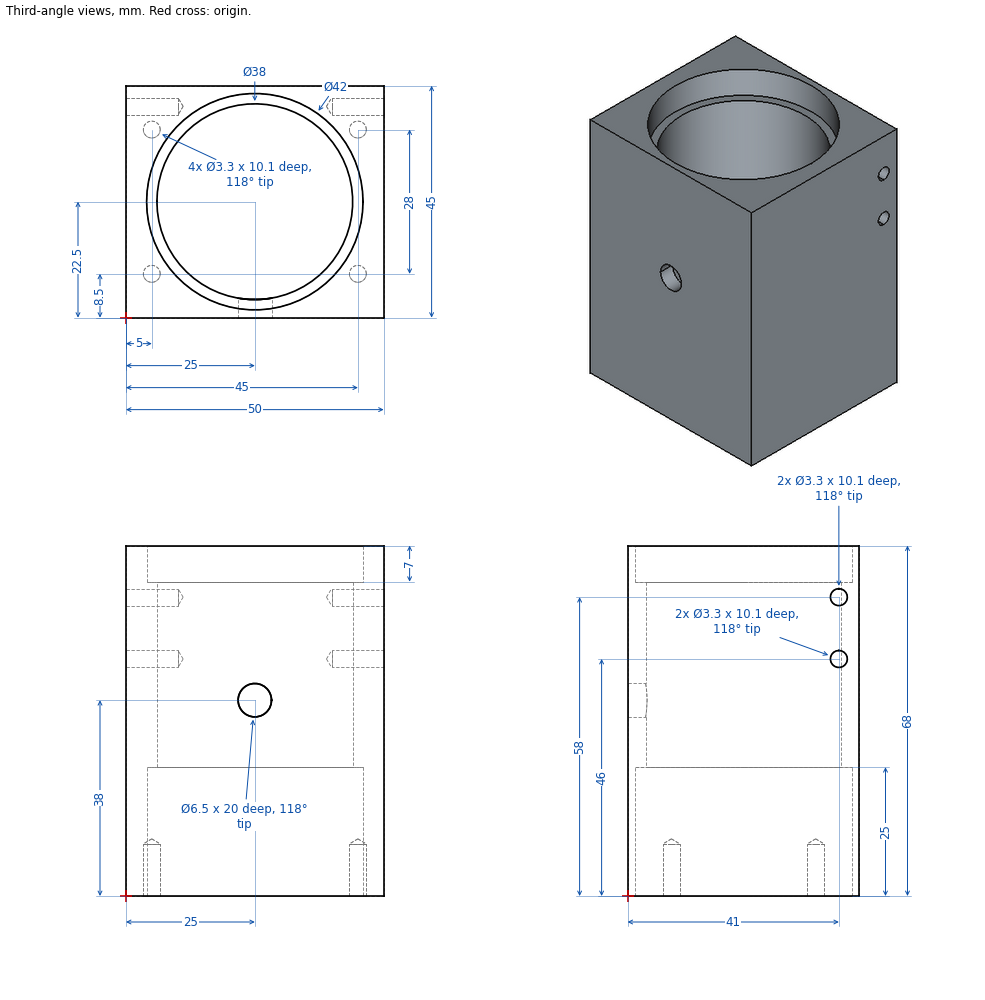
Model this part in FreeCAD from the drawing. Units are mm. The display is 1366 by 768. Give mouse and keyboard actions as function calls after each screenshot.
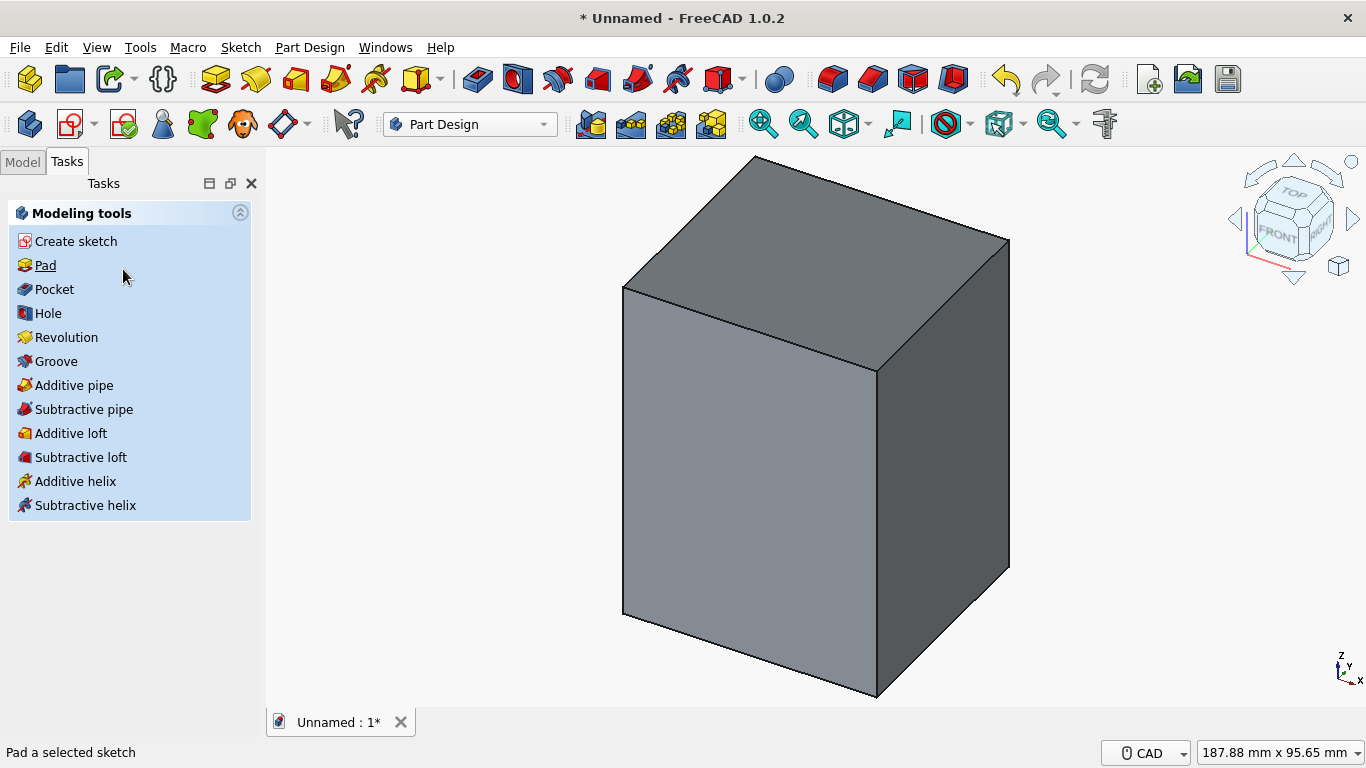
click(478, 80)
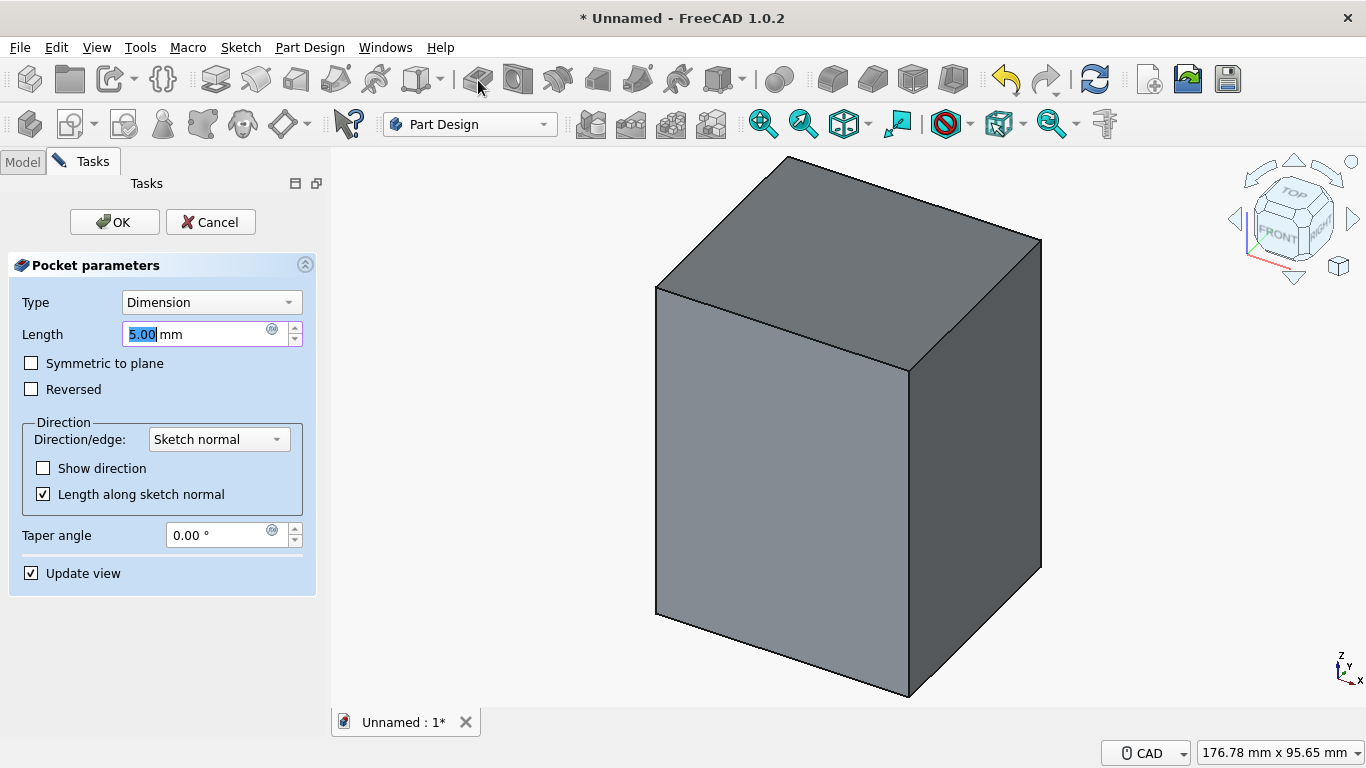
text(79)
key(Tab)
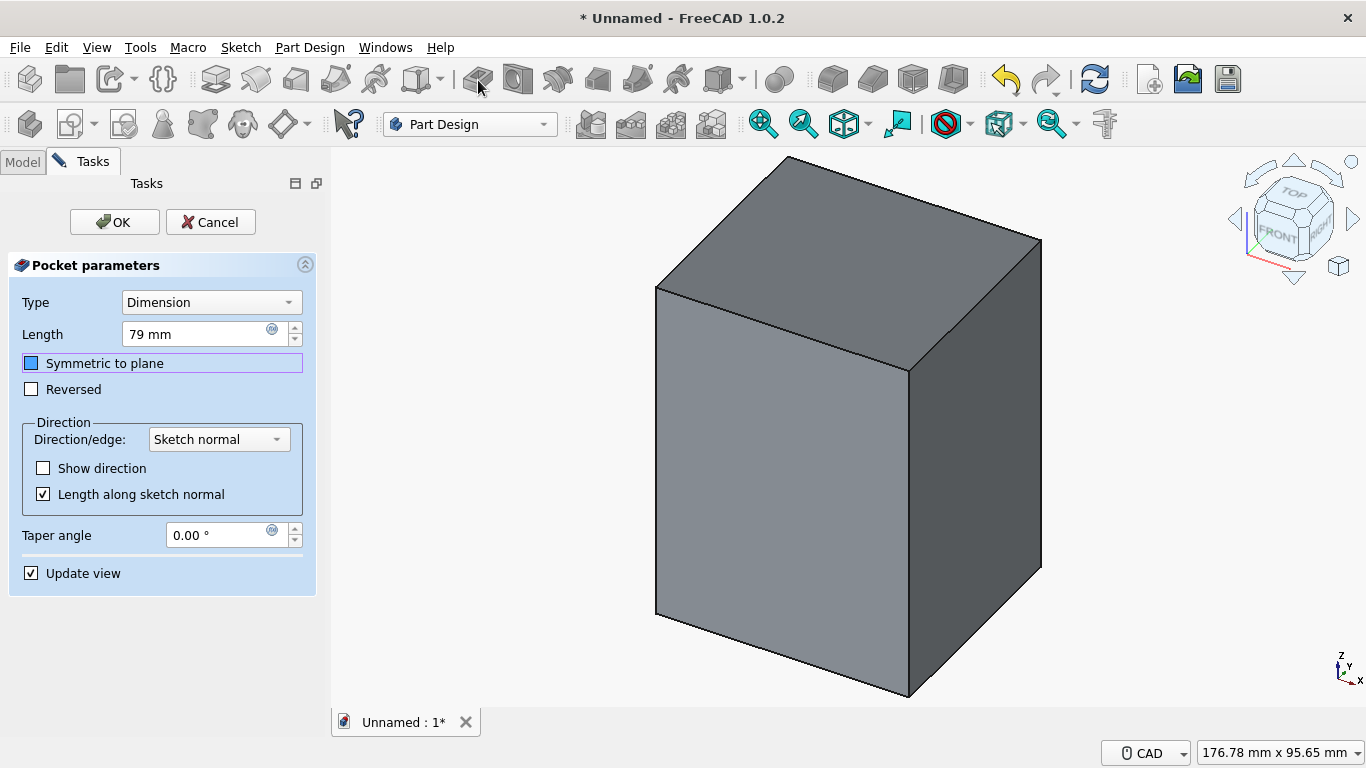
click(30, 389)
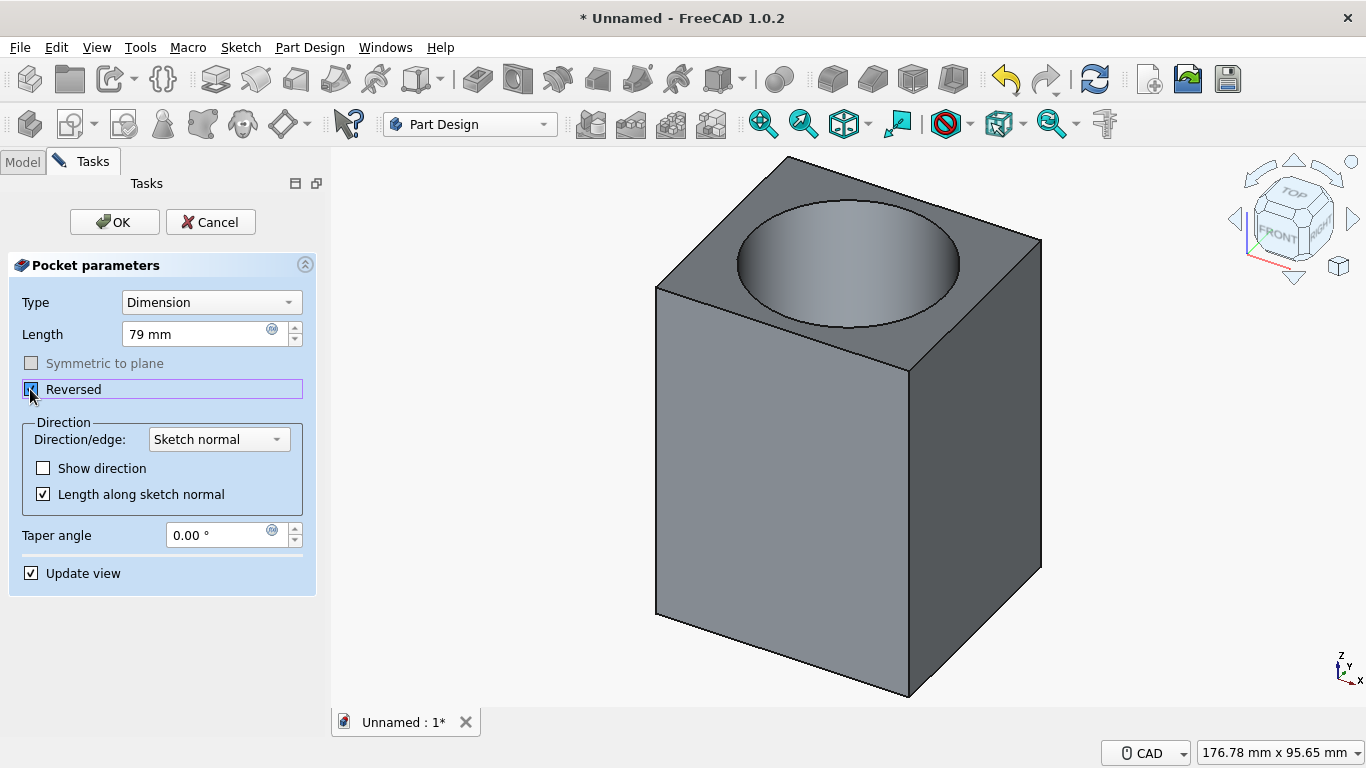
click(115, 222)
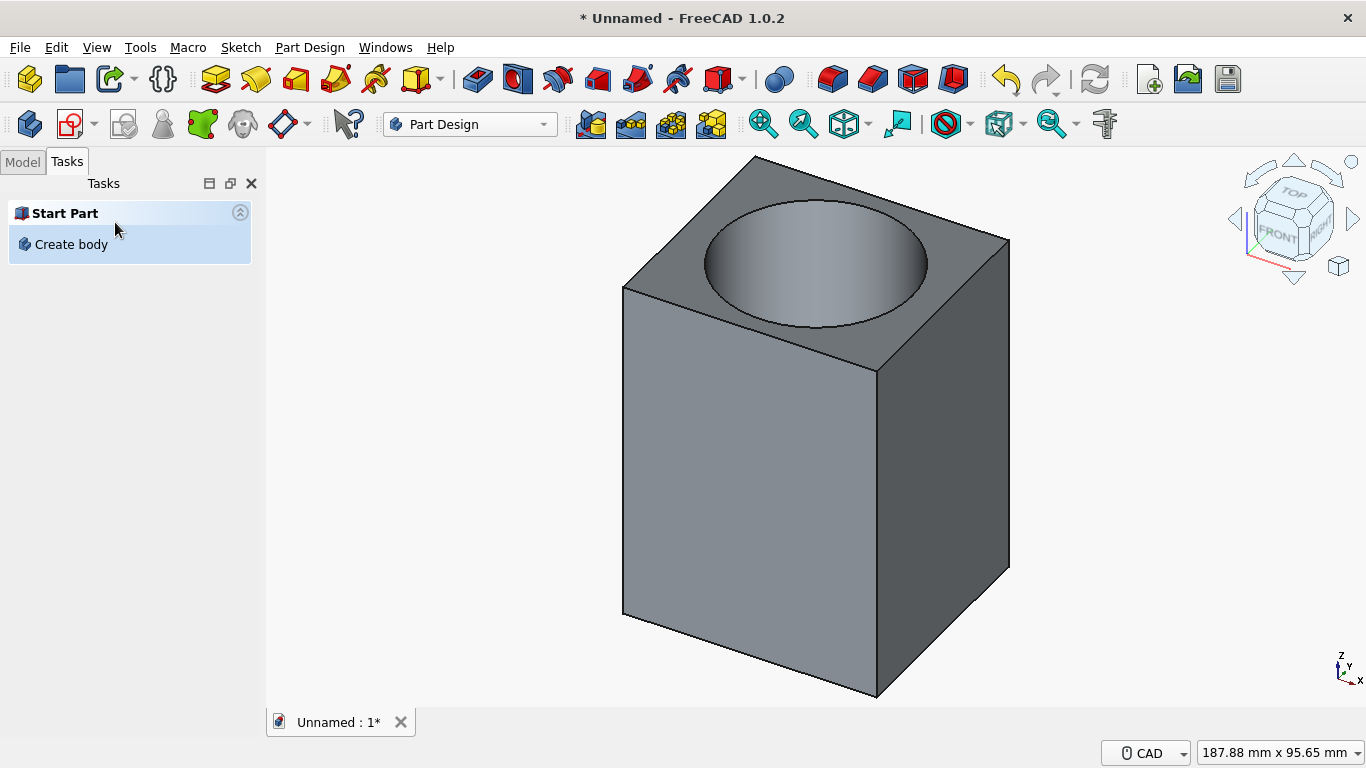
click(745, 190)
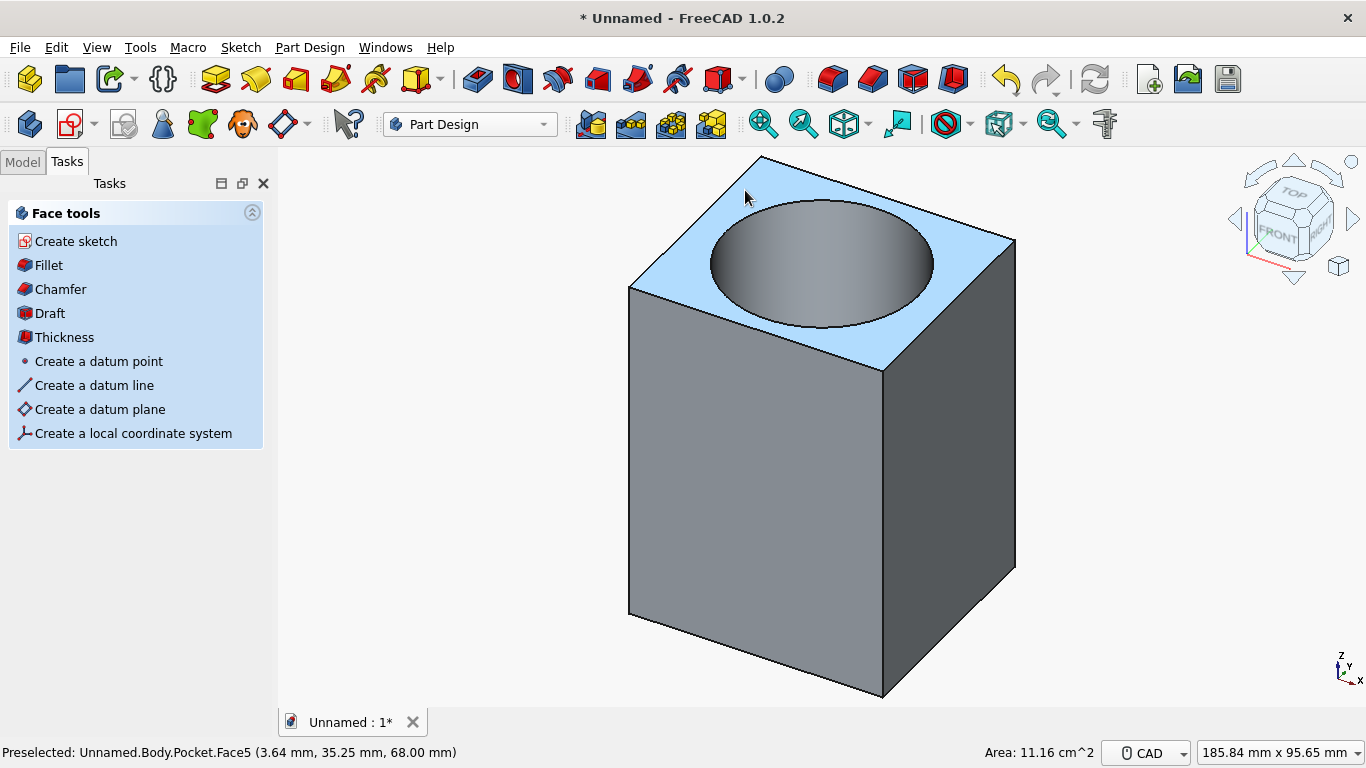
click(70, 124)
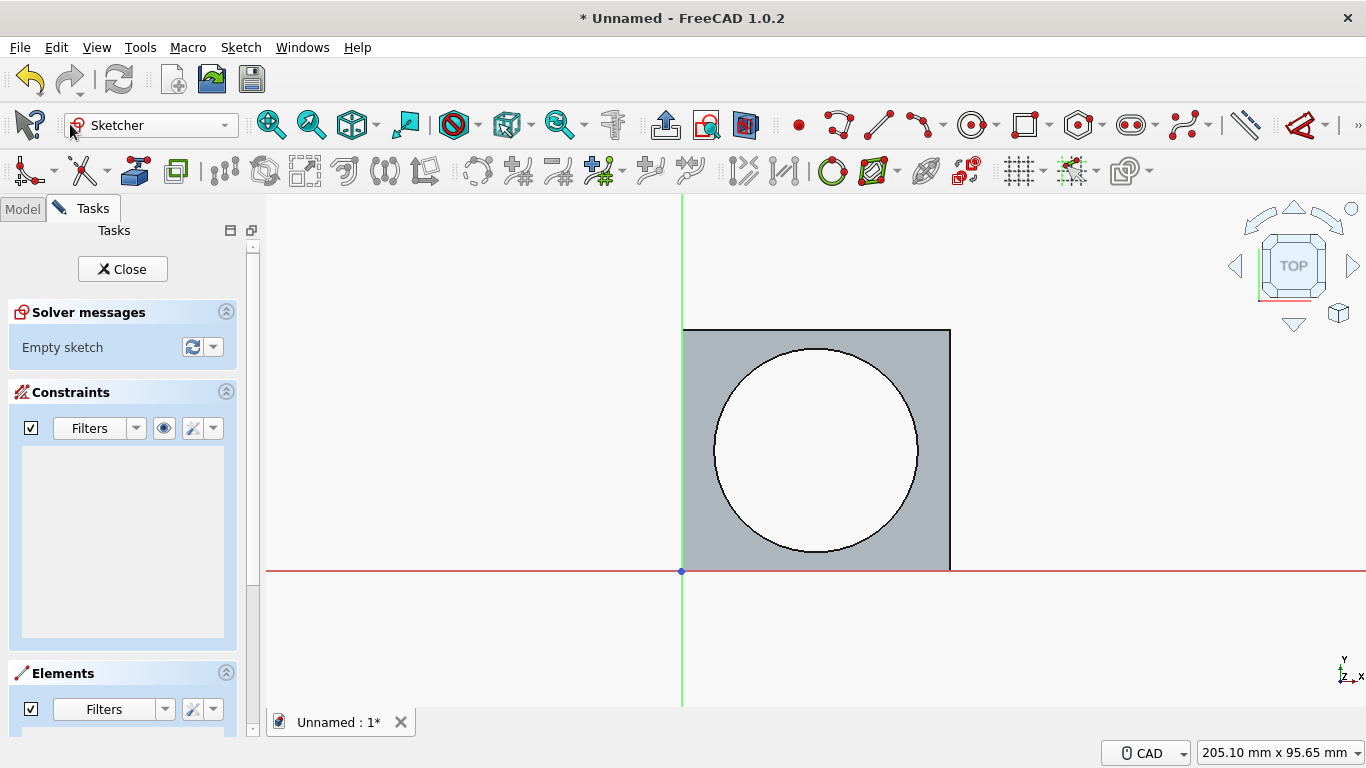
scroll(923, 463, up, 2)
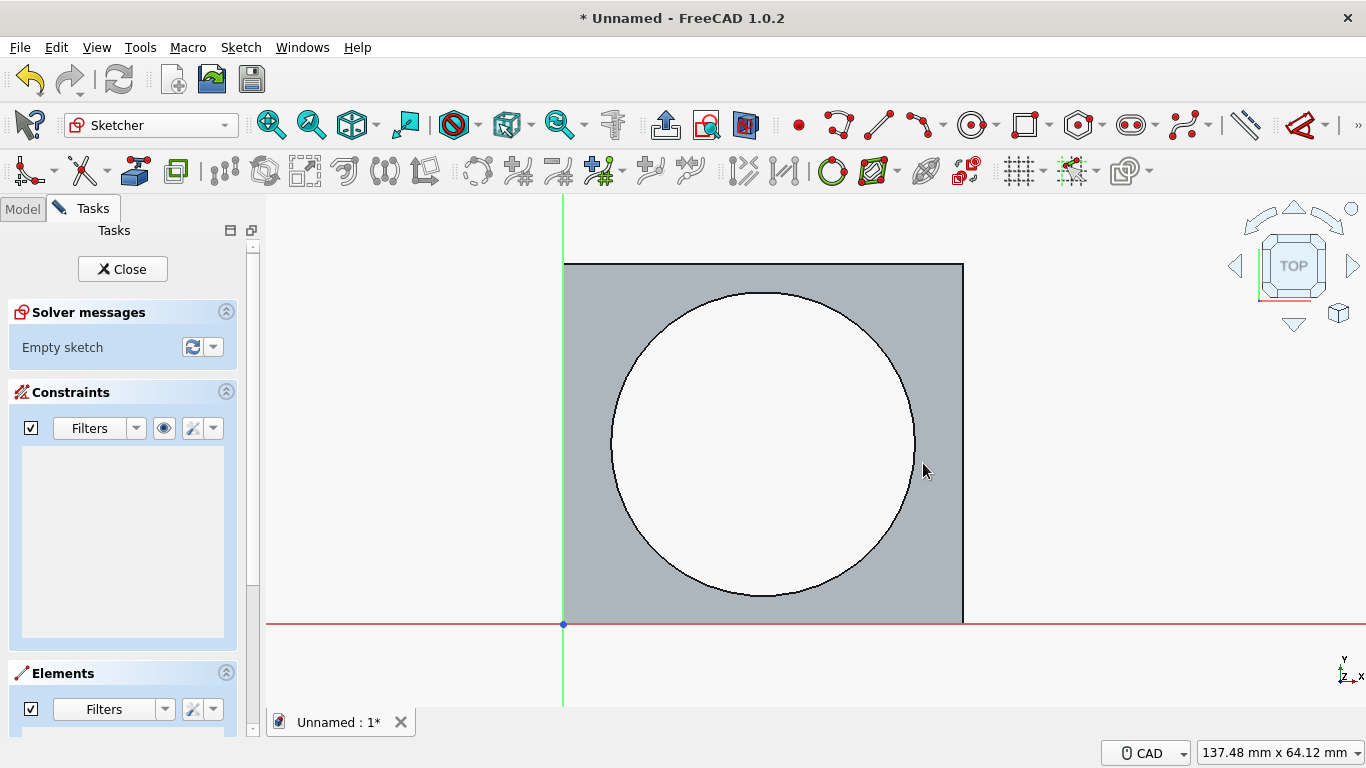
key(g)
key(c)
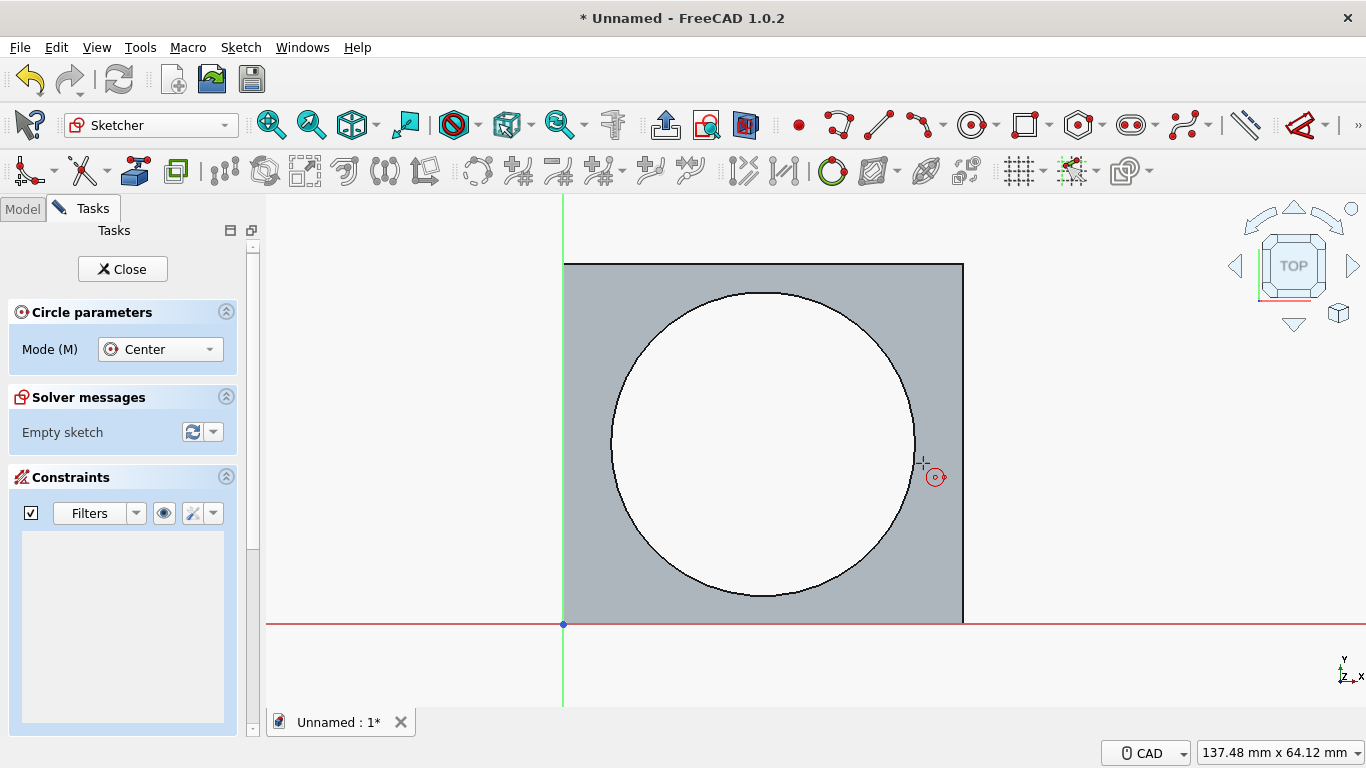
click(763, 444)
move(882, 325)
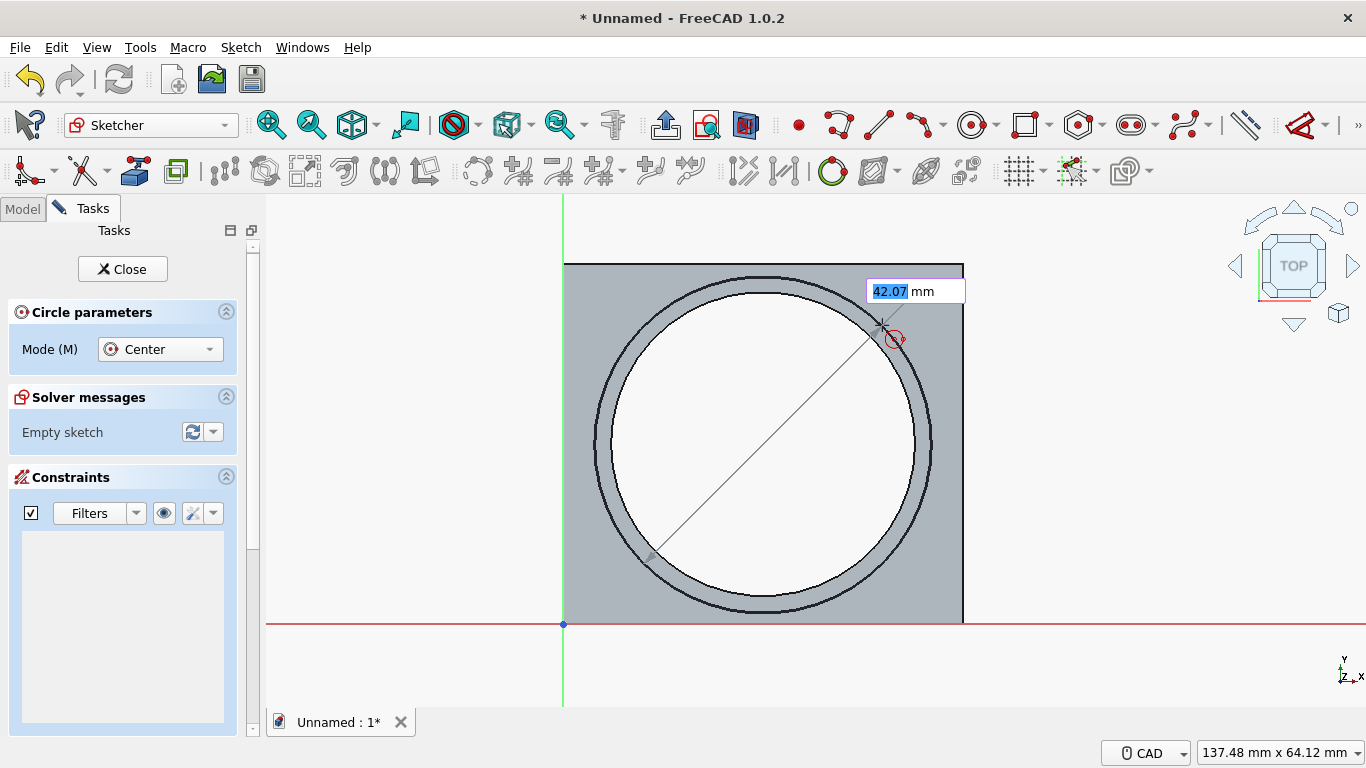
text(42)
key(Return)
key(Escape)